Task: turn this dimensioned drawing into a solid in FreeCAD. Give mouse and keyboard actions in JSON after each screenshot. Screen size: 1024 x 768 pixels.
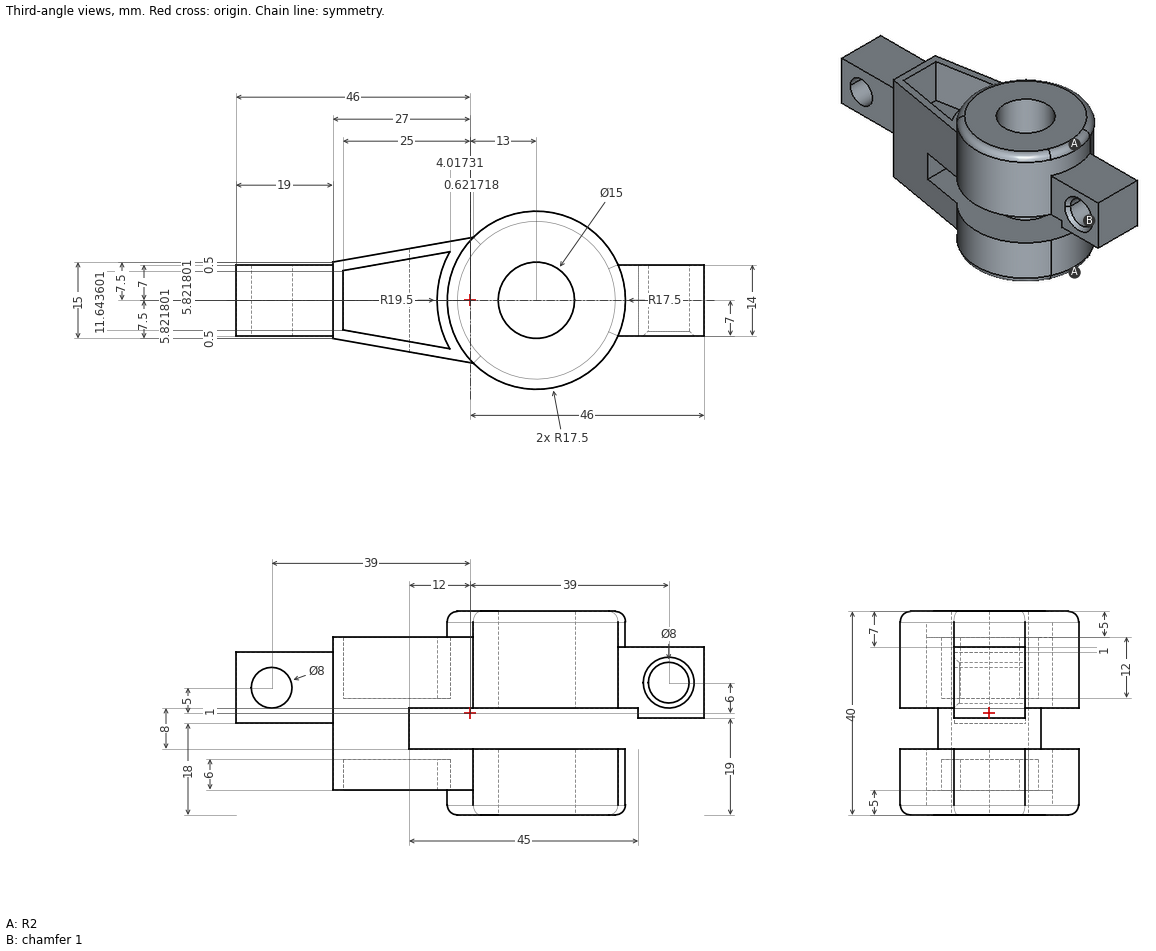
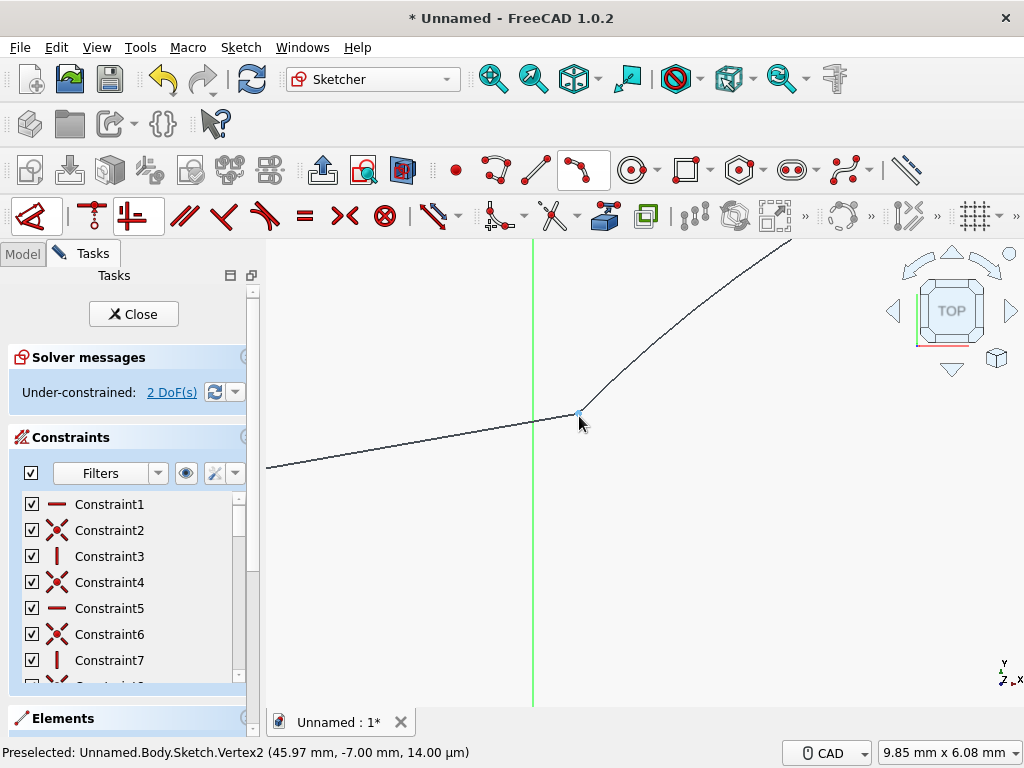
{"action": "left_click", "coordinate": [578, 414]}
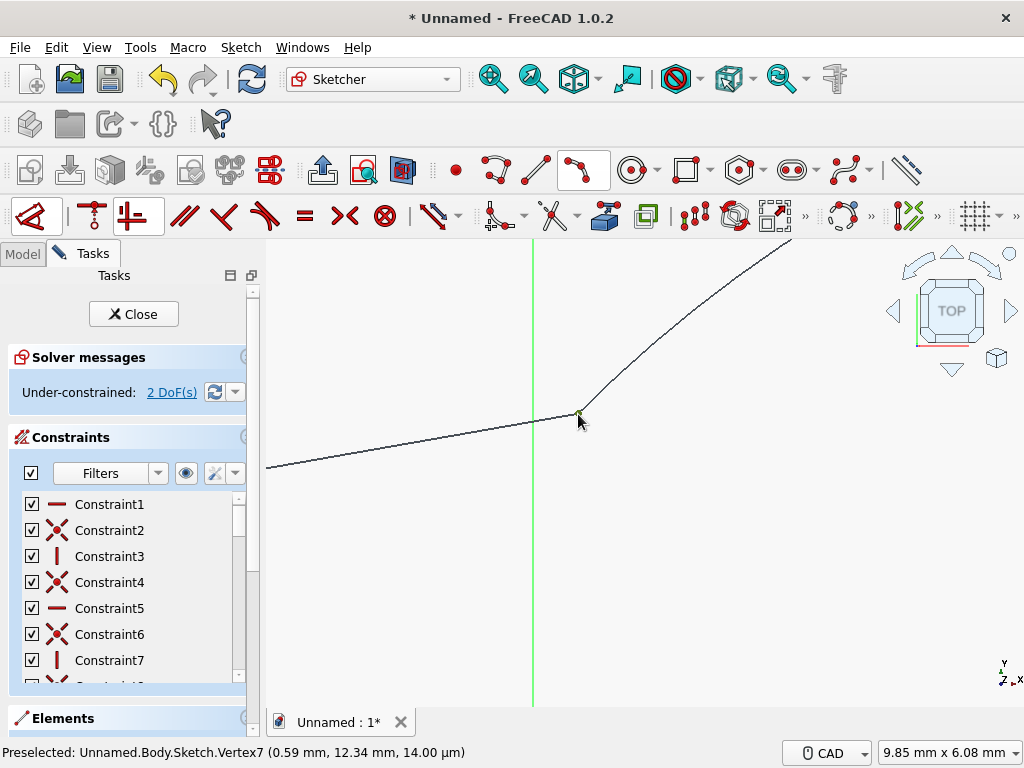
{"action": "left_click", "coordinate": [56, 216]}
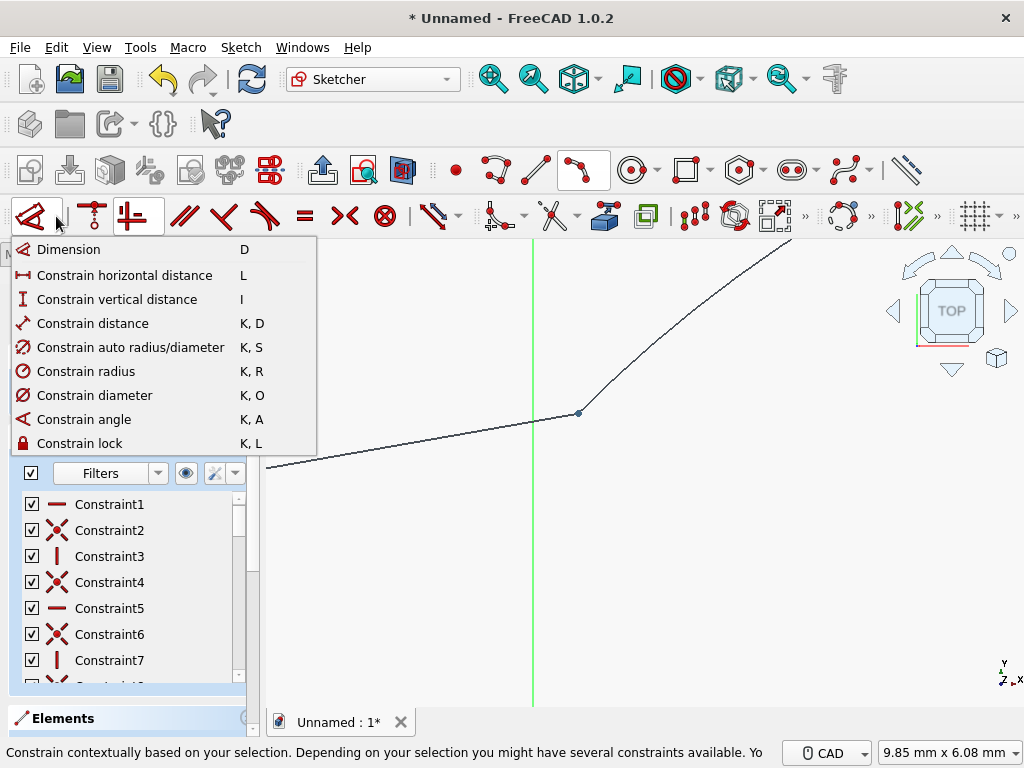
{"action": "left_click", "coordinate": [164, 275]}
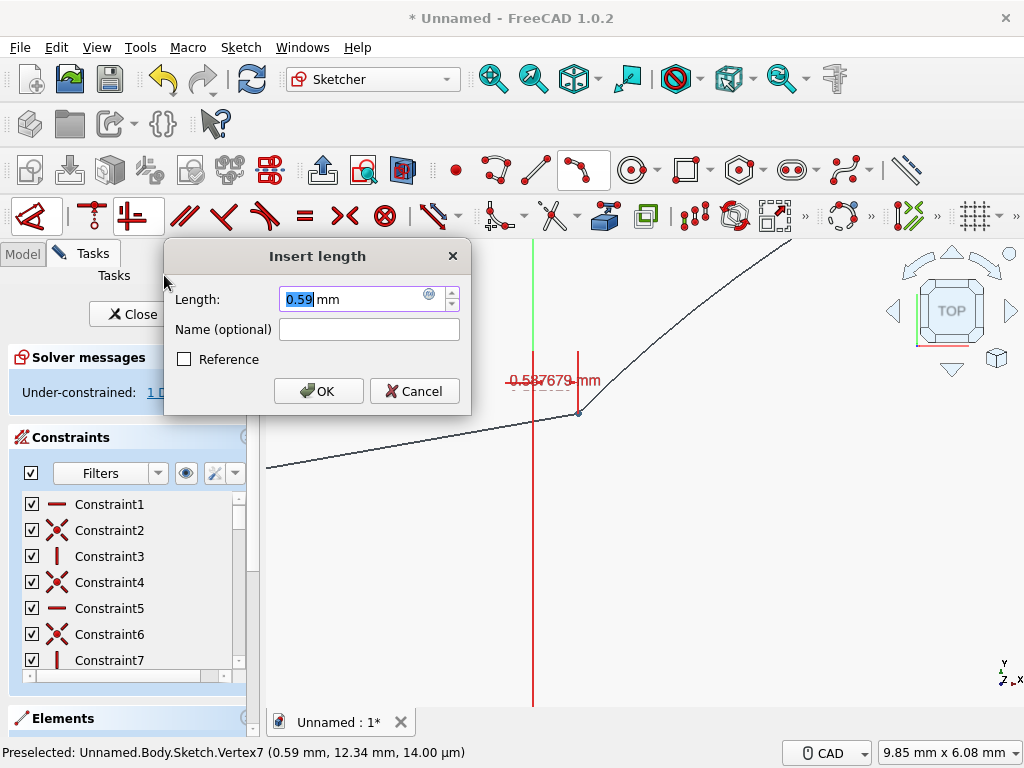
{"action": "type", "text": "0.621718"}
{"action": "key", "text": "Return"}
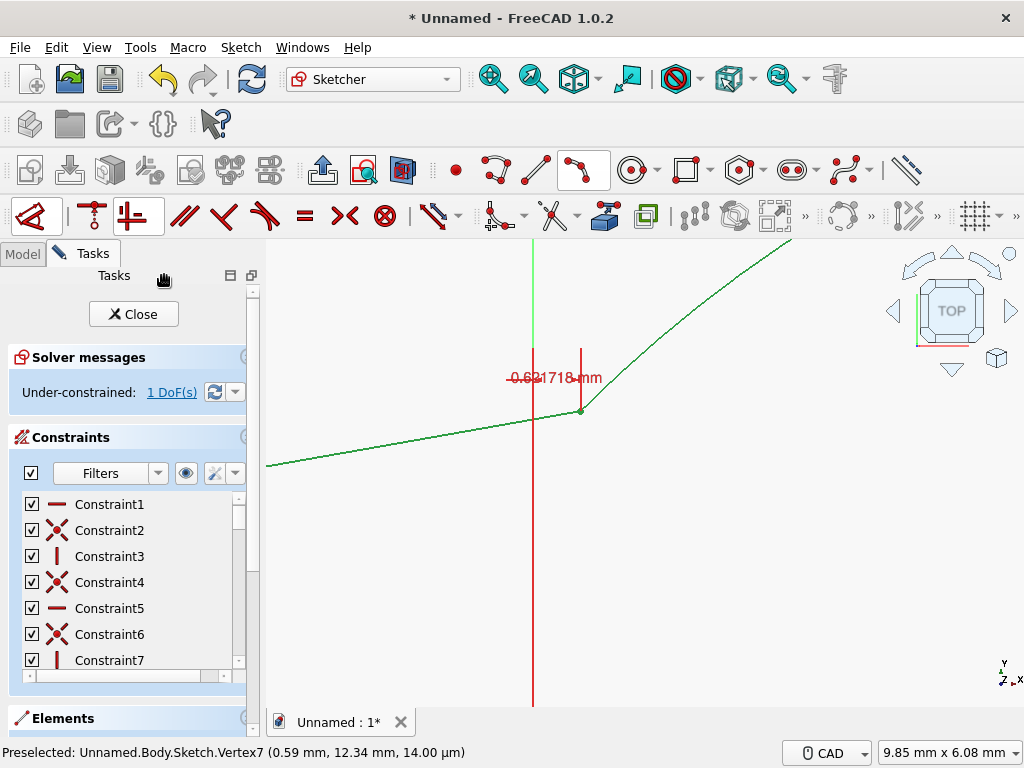
{"action": "scroll", "coordinate": [579, 415], "scroll_direction": "down", "scroll_amount": 14}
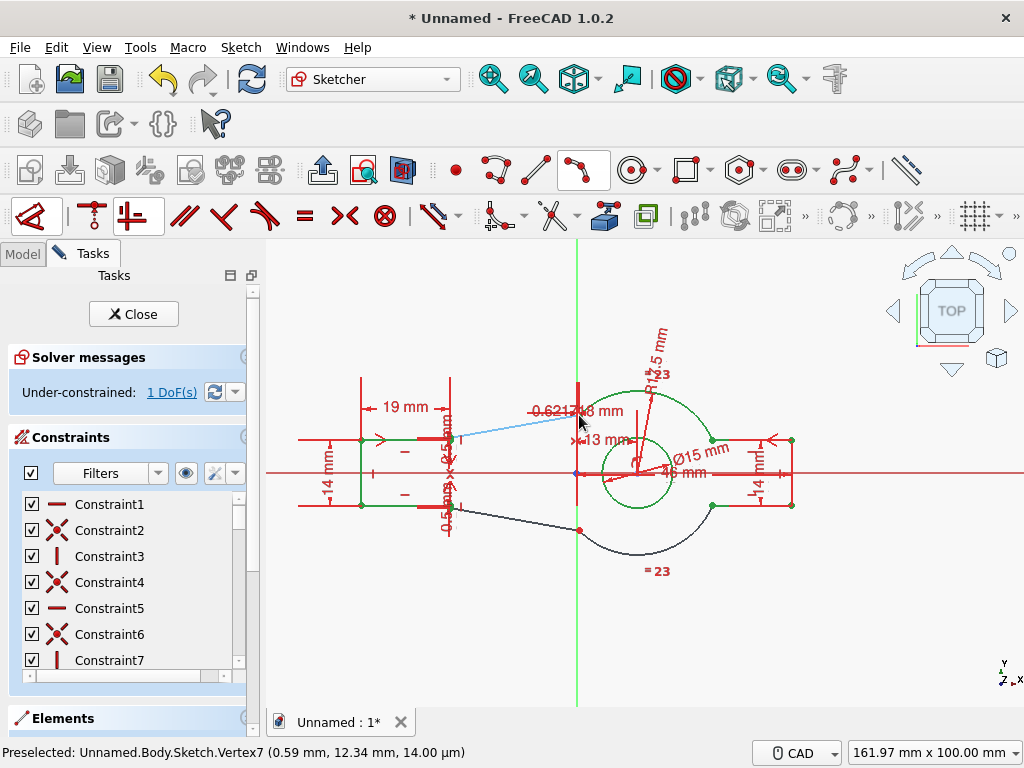
{"action": "scroll", "coordinate": [579, 531], "scroll_direction": "up", "scroll_amount": 14}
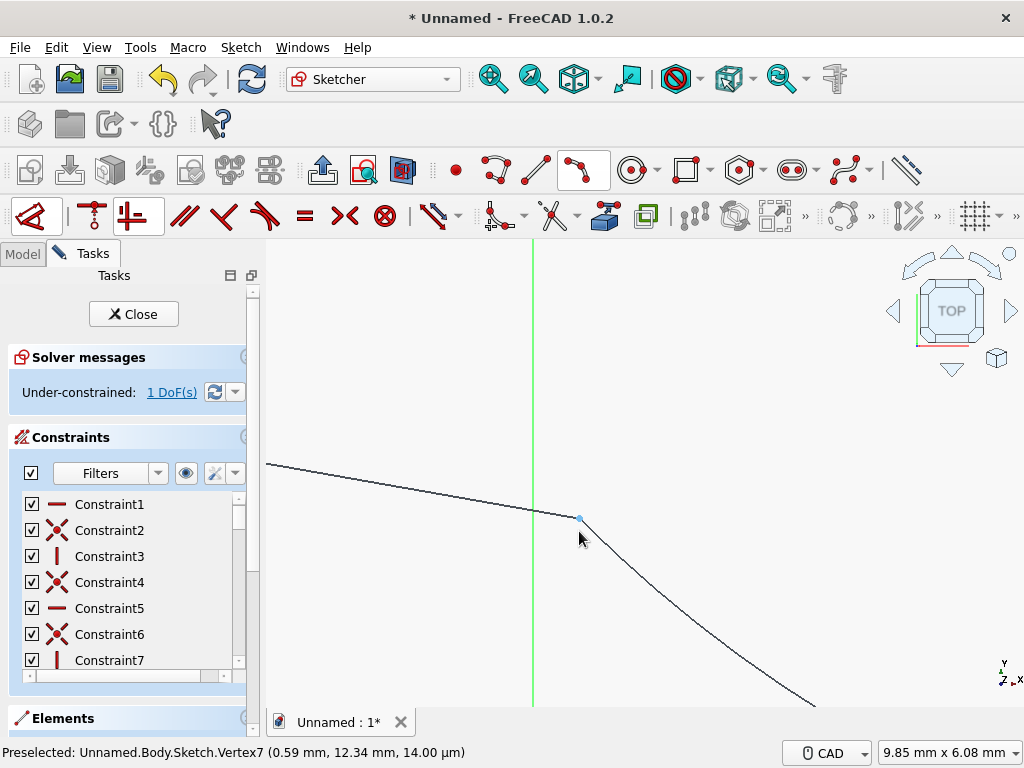
{"action": "left_click", "coordinate": [580, 519]}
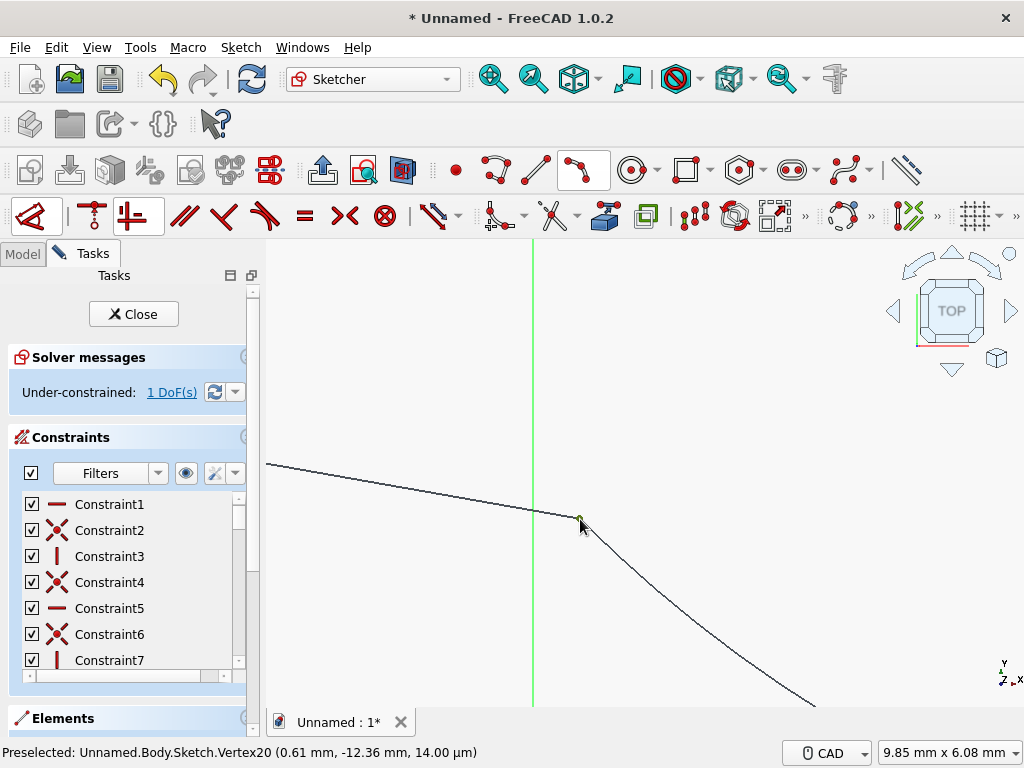
{"action": "key", "text": "l"}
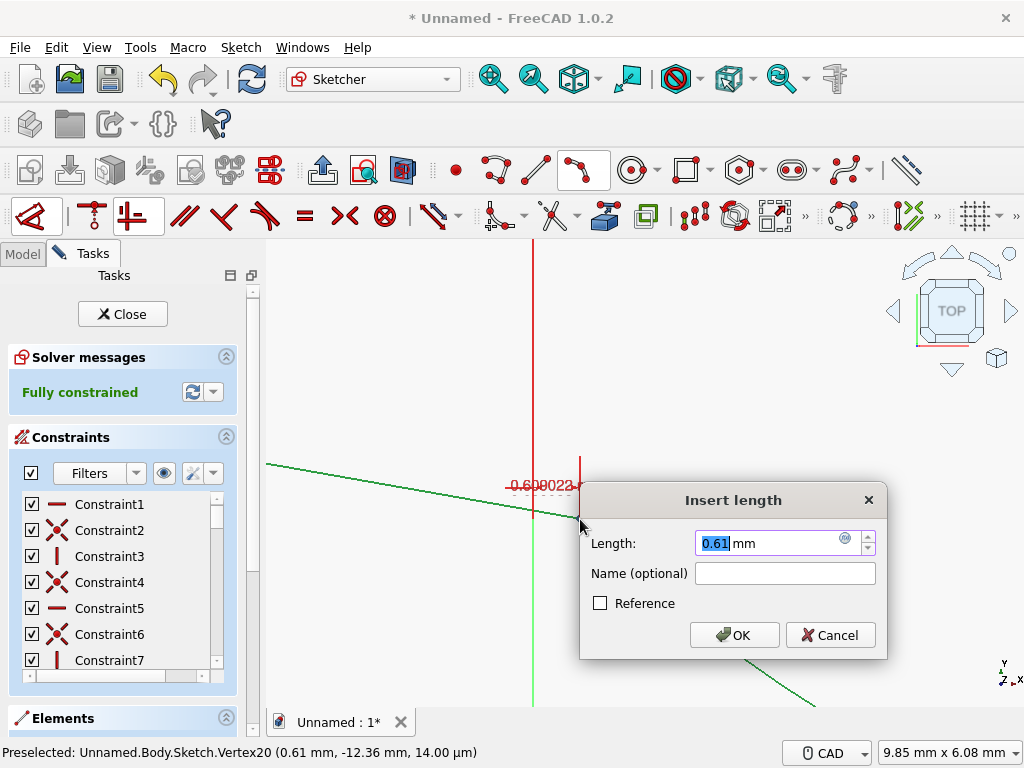
{"action": "type", "text": "0.621718"}
{"action": "key", "text": "Return"}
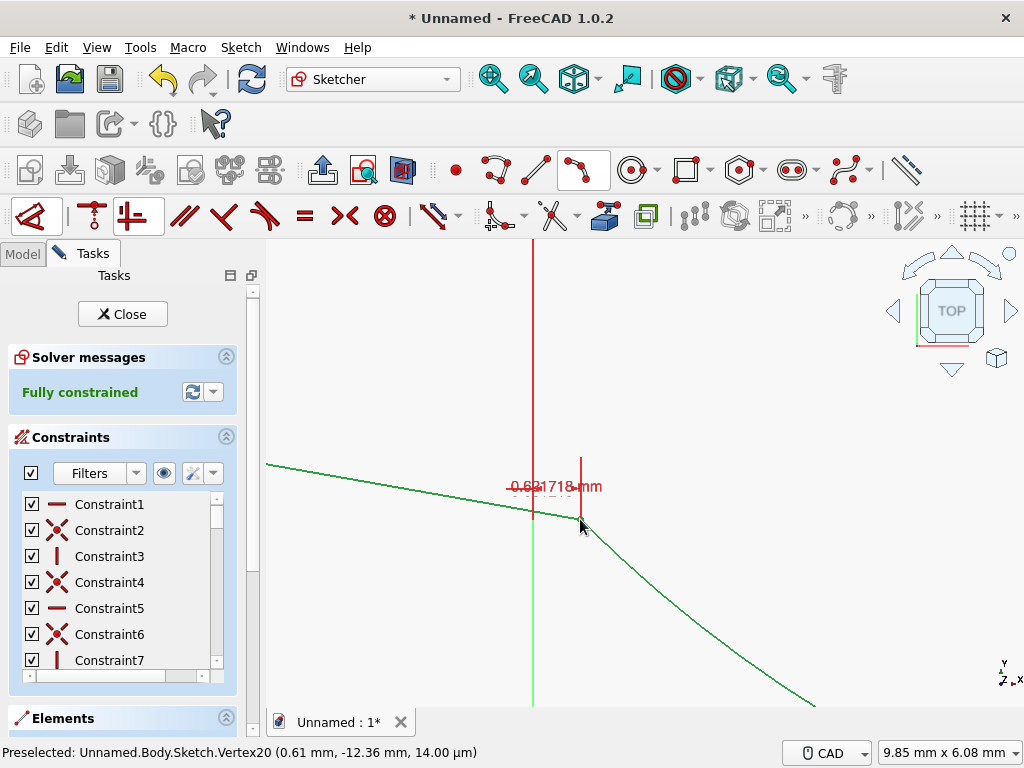
{"action": "left_click", "coordinate": [123, 314]}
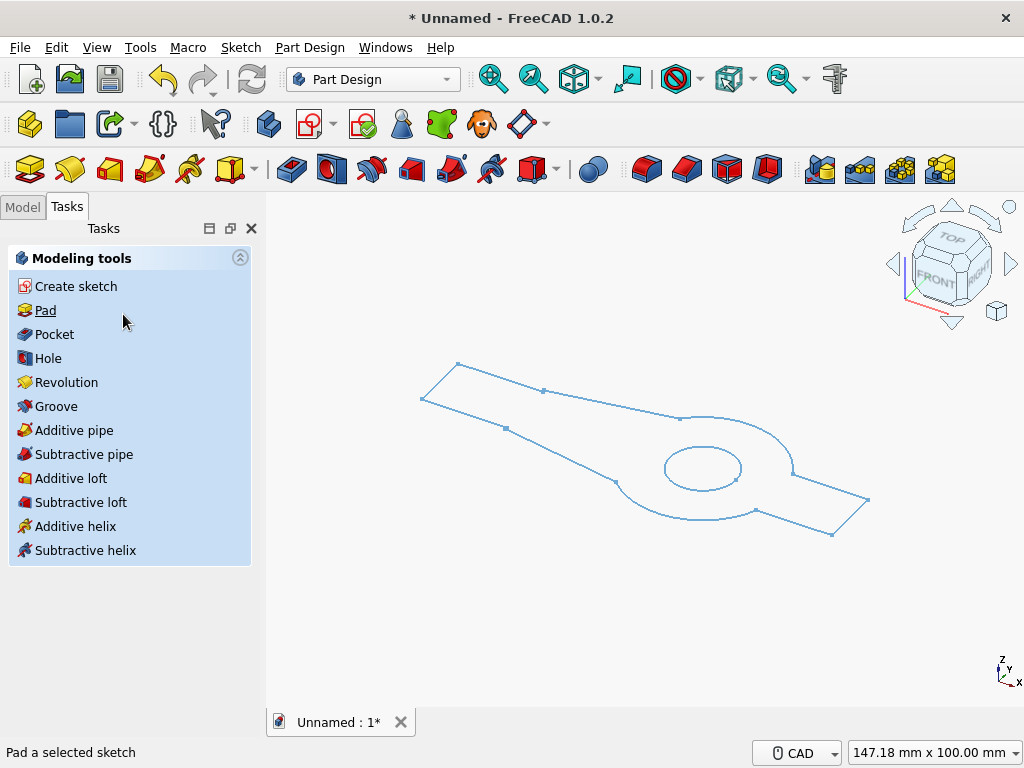
{"action": "left_click", "coordinate": [30, 170]}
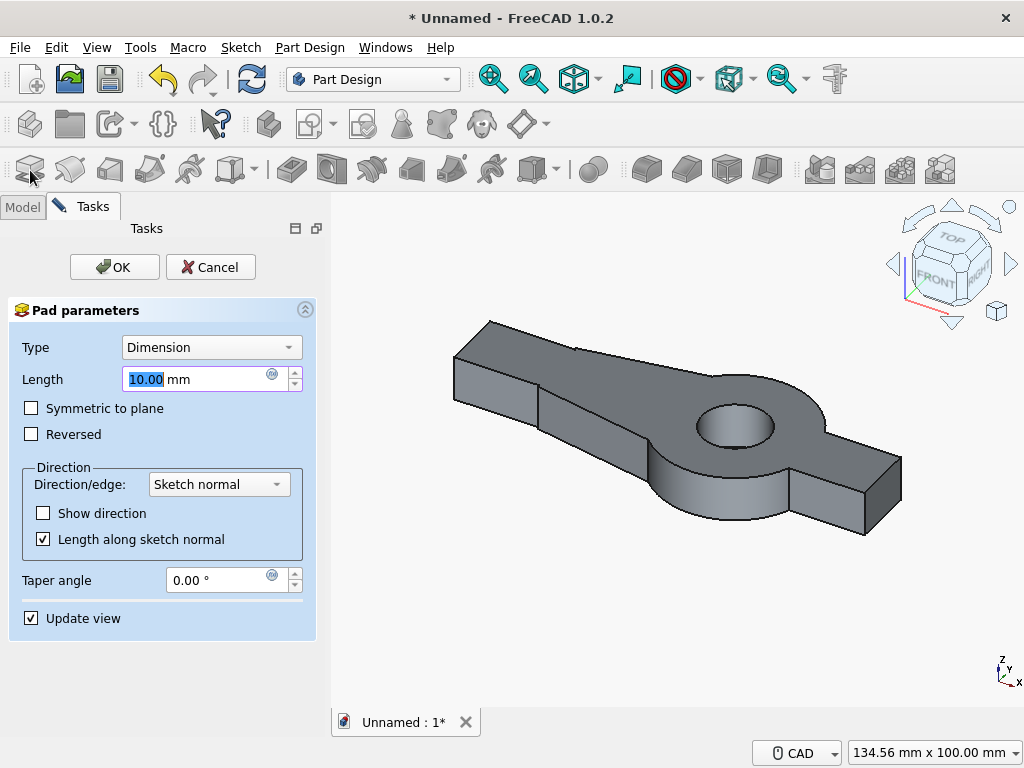
{"action": "type", "text": "40"}
{"action": "key", "text": "Tab"}